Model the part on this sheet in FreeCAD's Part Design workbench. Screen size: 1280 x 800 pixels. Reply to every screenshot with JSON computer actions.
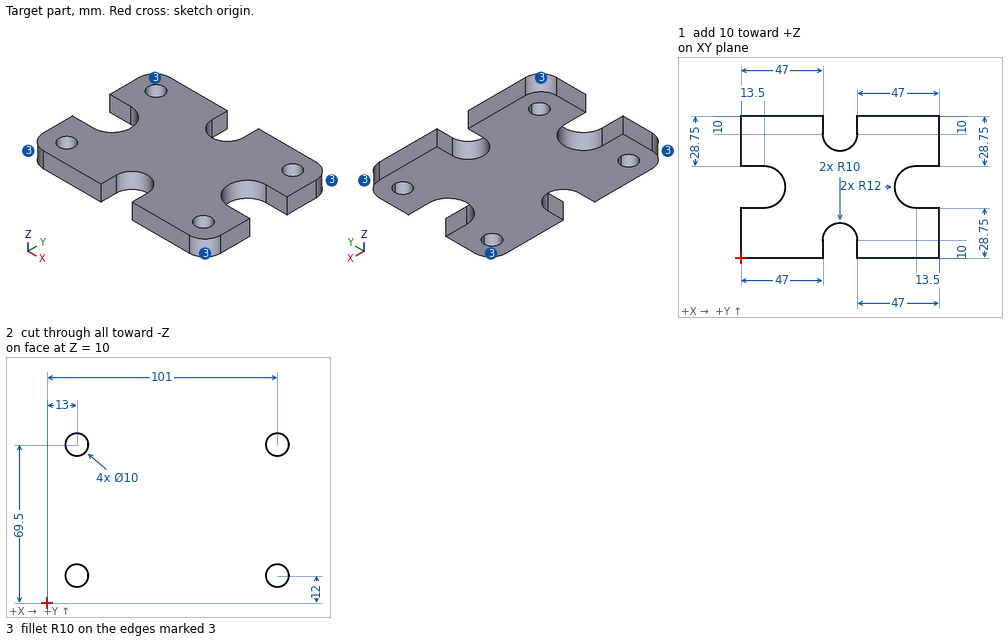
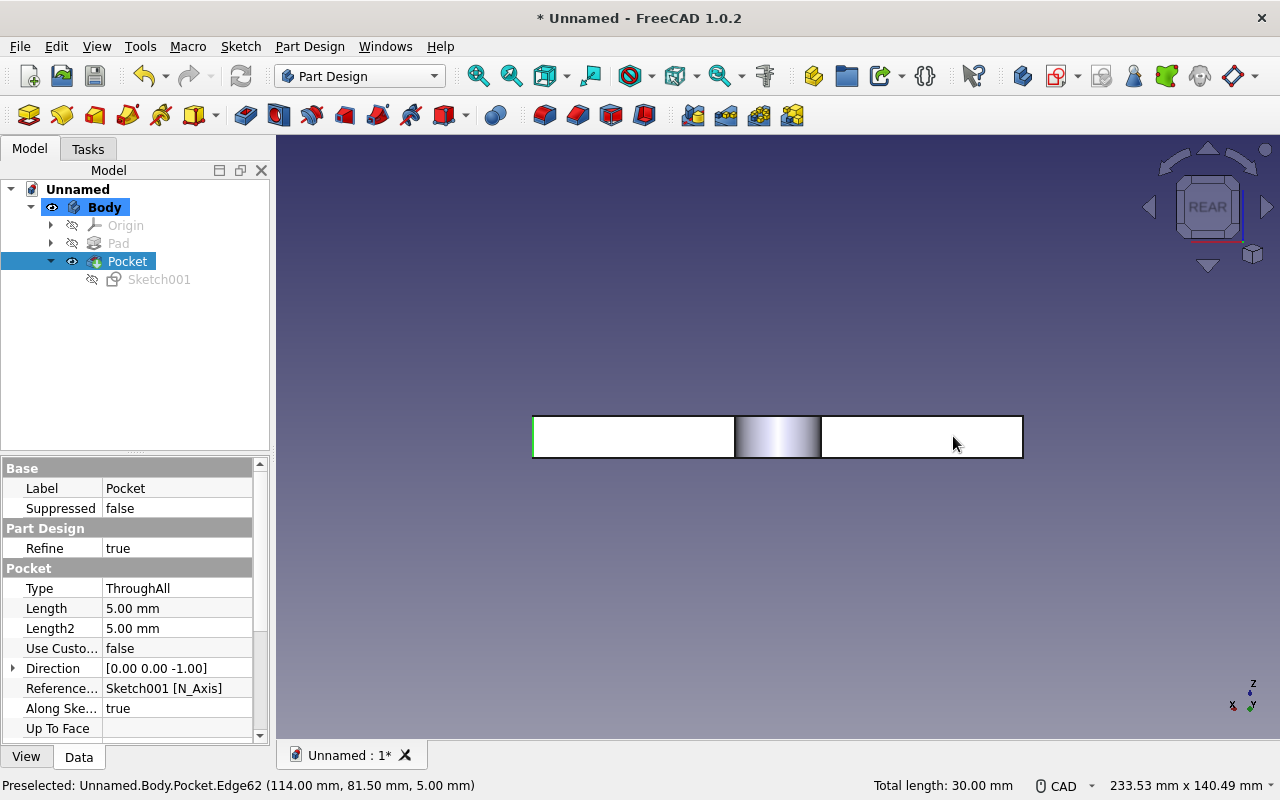
{"action": "left_click", "coordinate": [1023, 436], "text": "ctrl"}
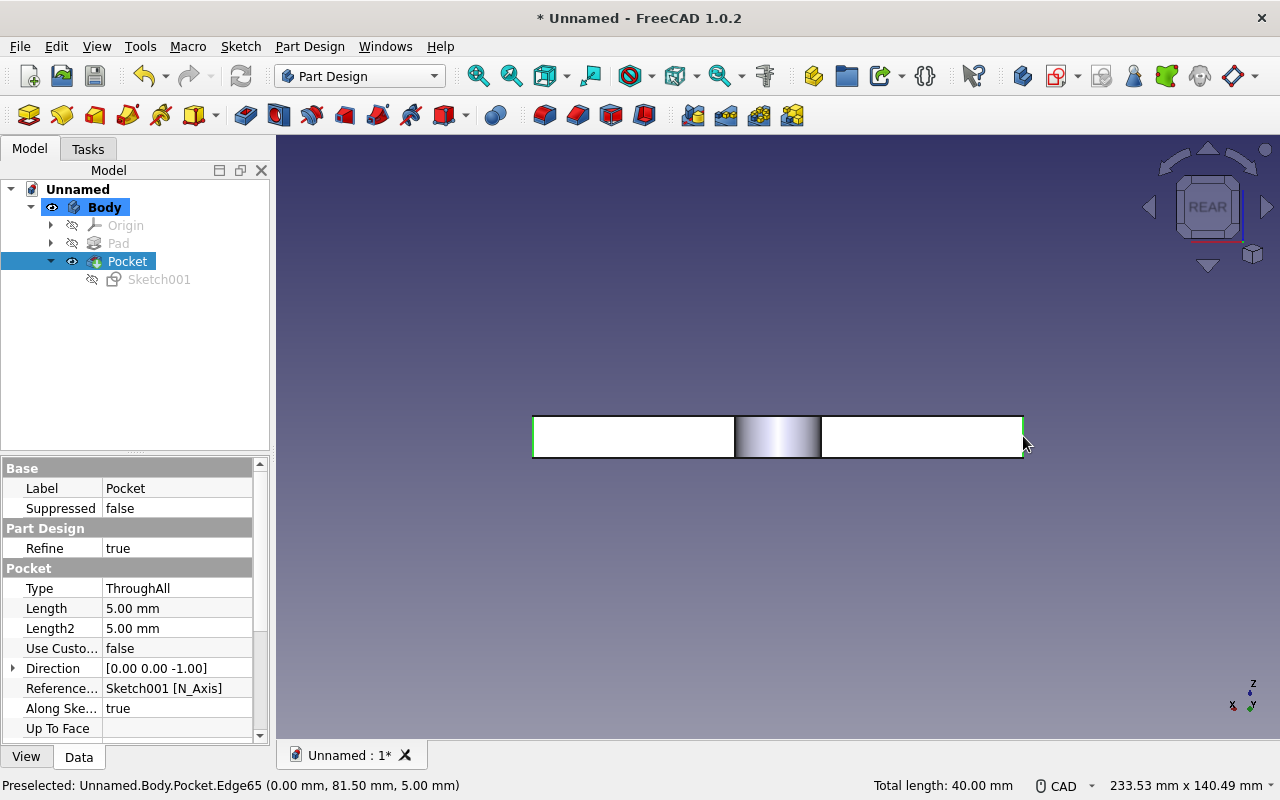
{"action": "left_click", "coordinate": [545, 116]}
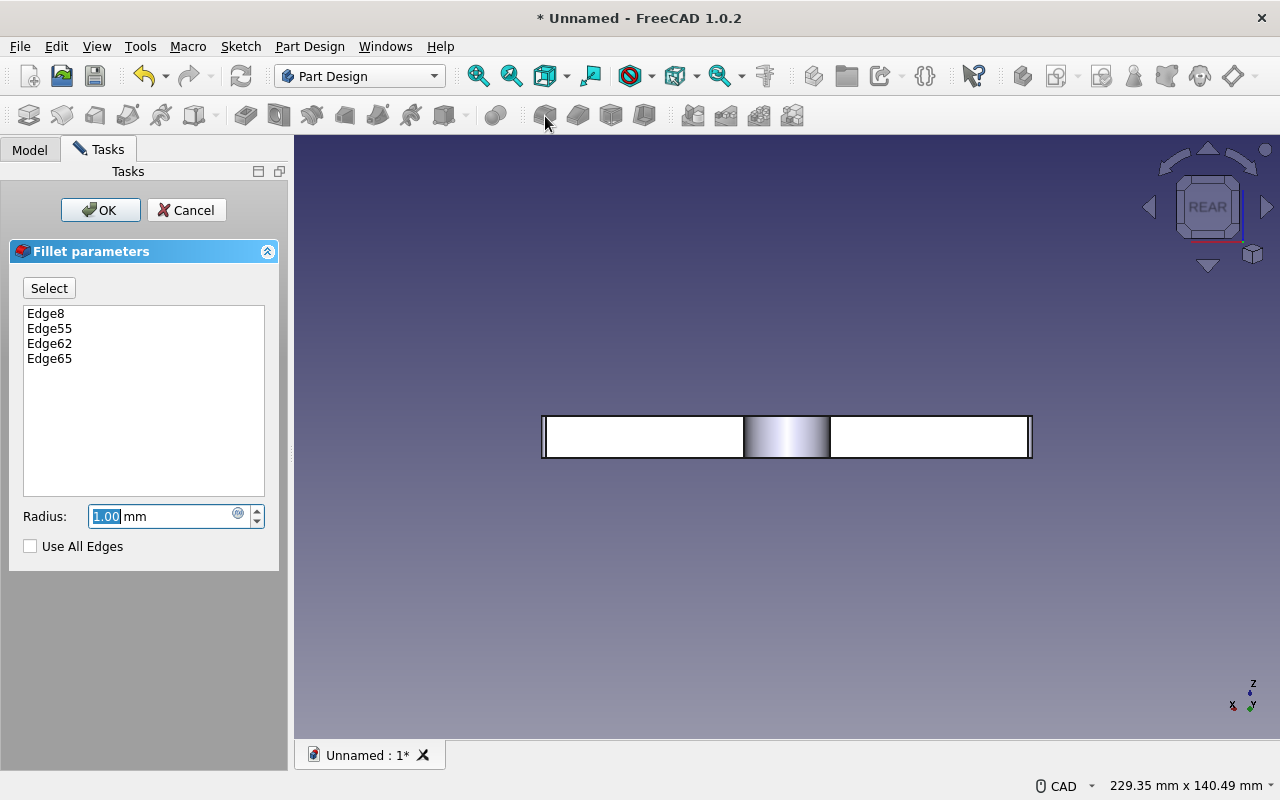
{"action": "type", "text": "10"}
{"action": "key", "text": "Tab"}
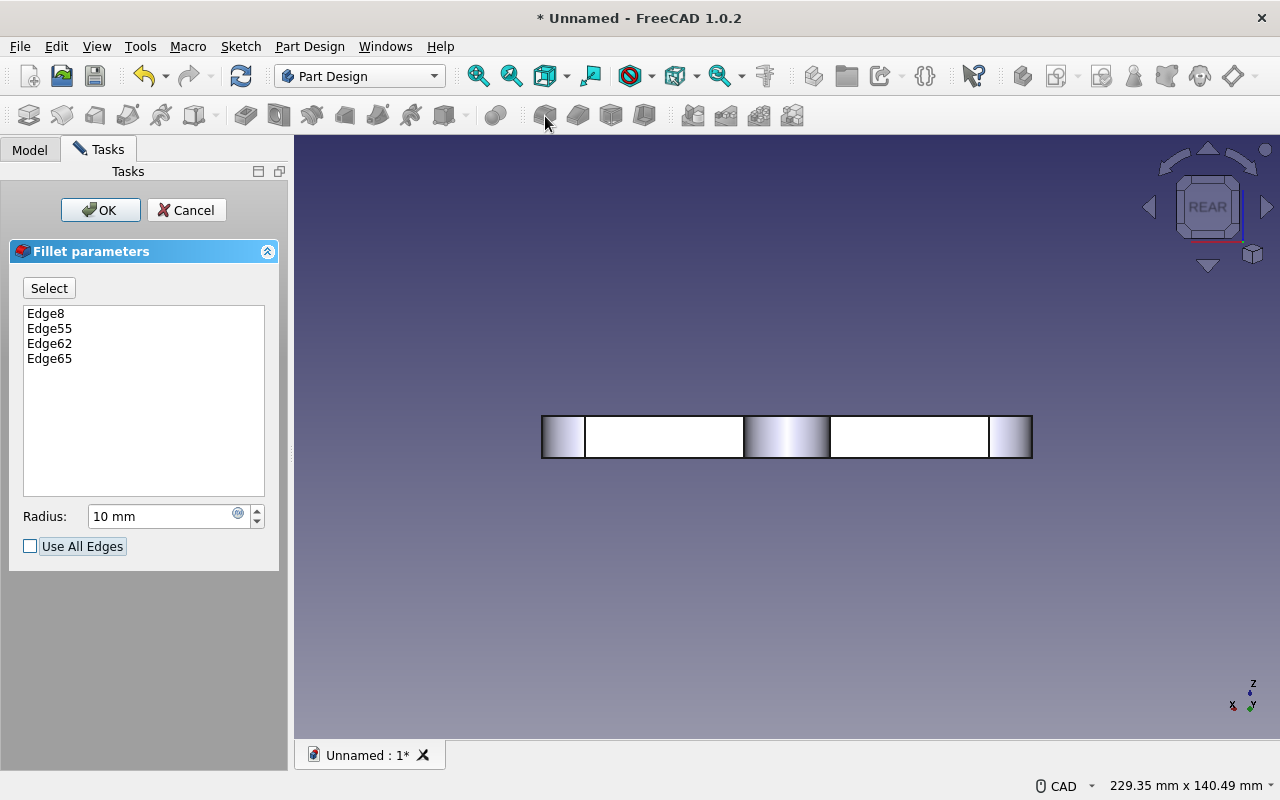
{"action": "left_click", "coordinate": [101, 210]}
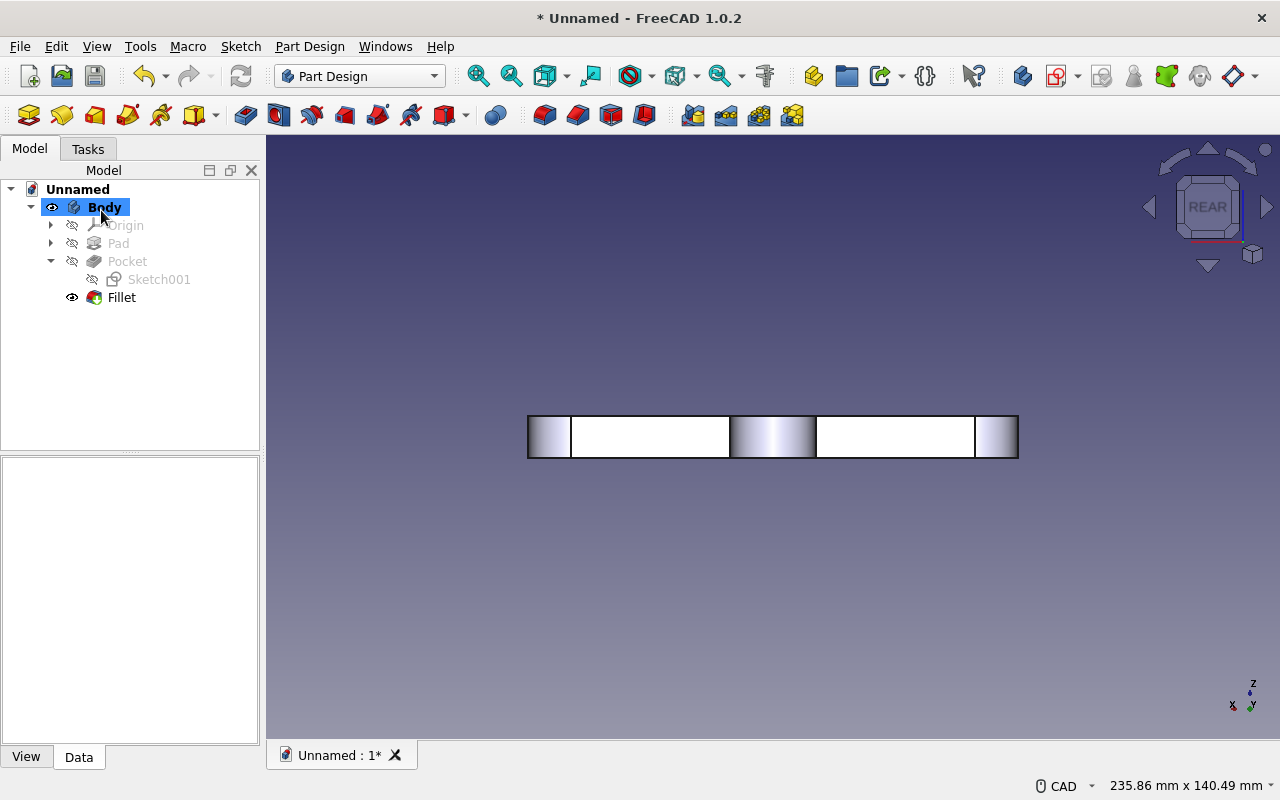
{"action": "key", "text": "0"}